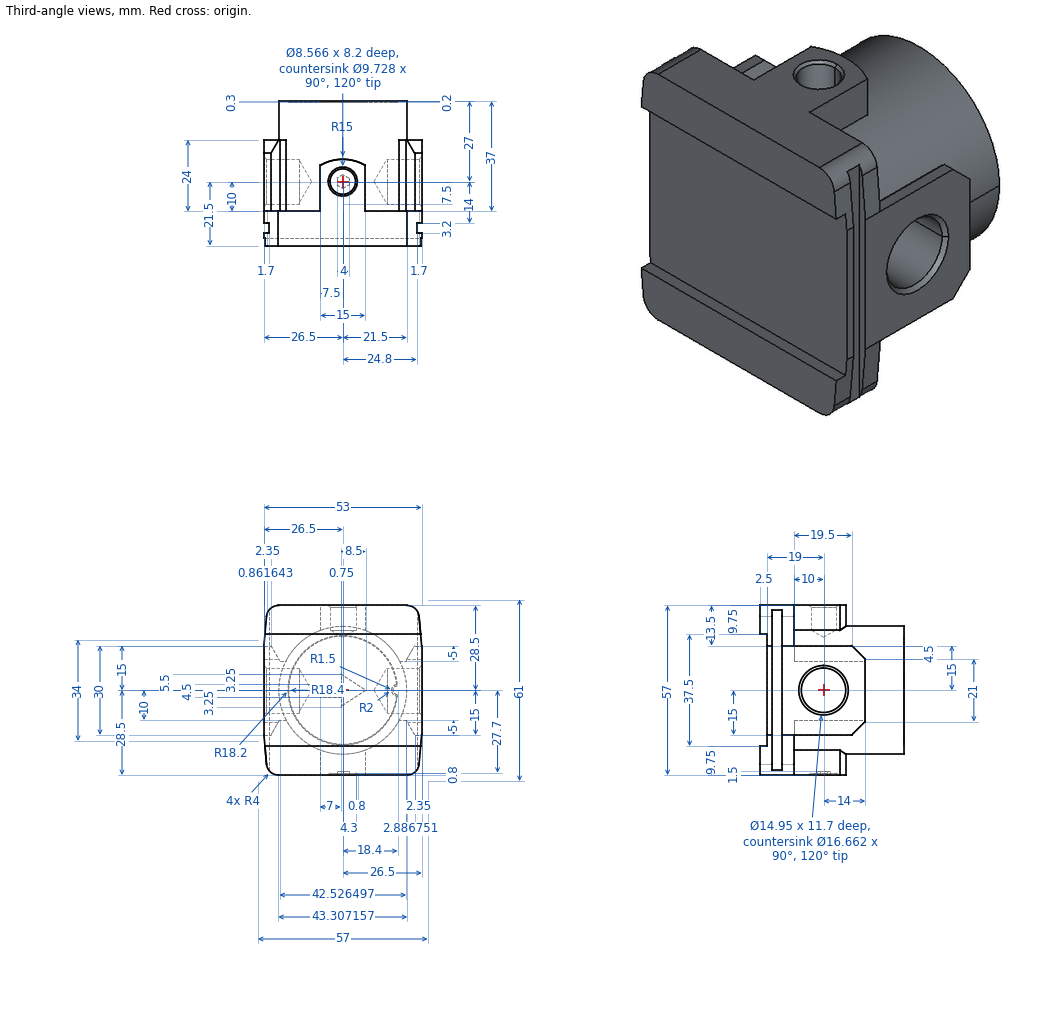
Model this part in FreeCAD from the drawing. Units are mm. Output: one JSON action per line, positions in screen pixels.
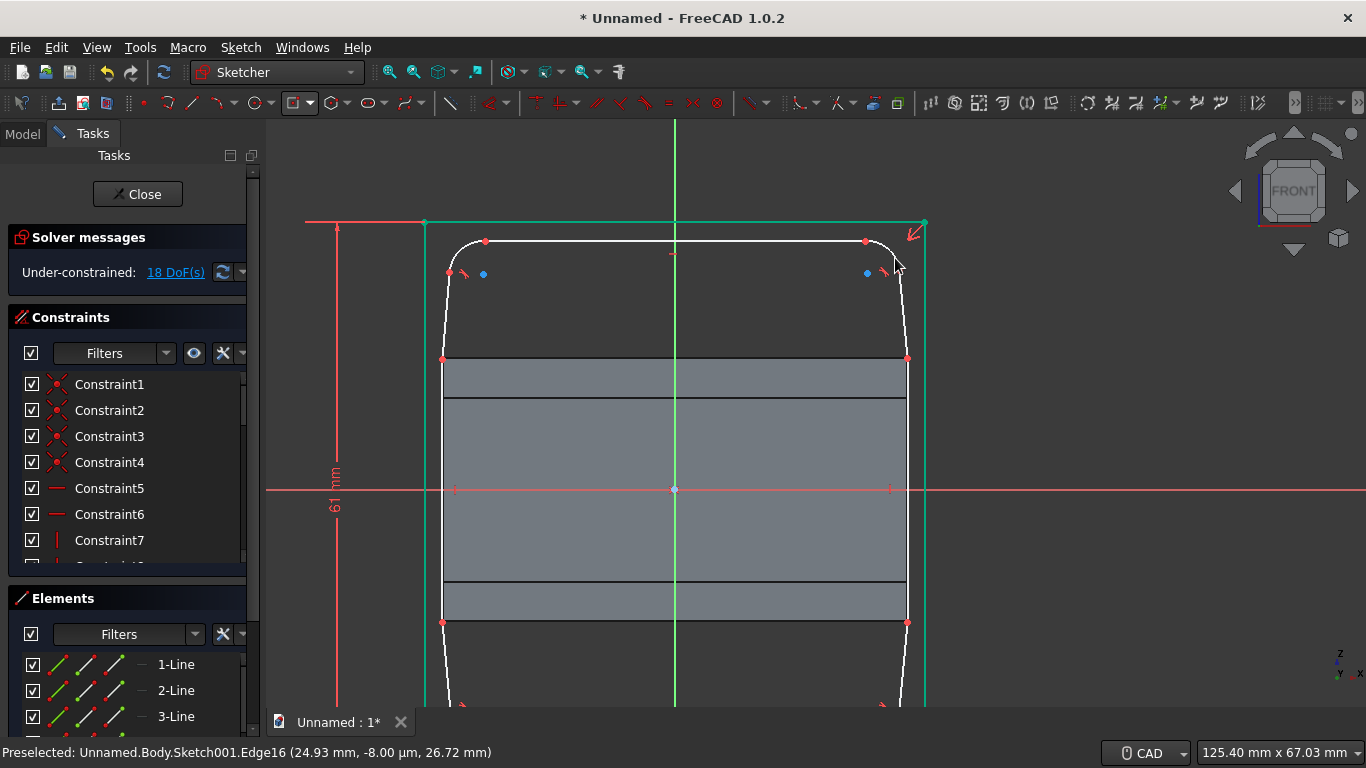
{"action": "left_click", "coordinate": [751, 241]}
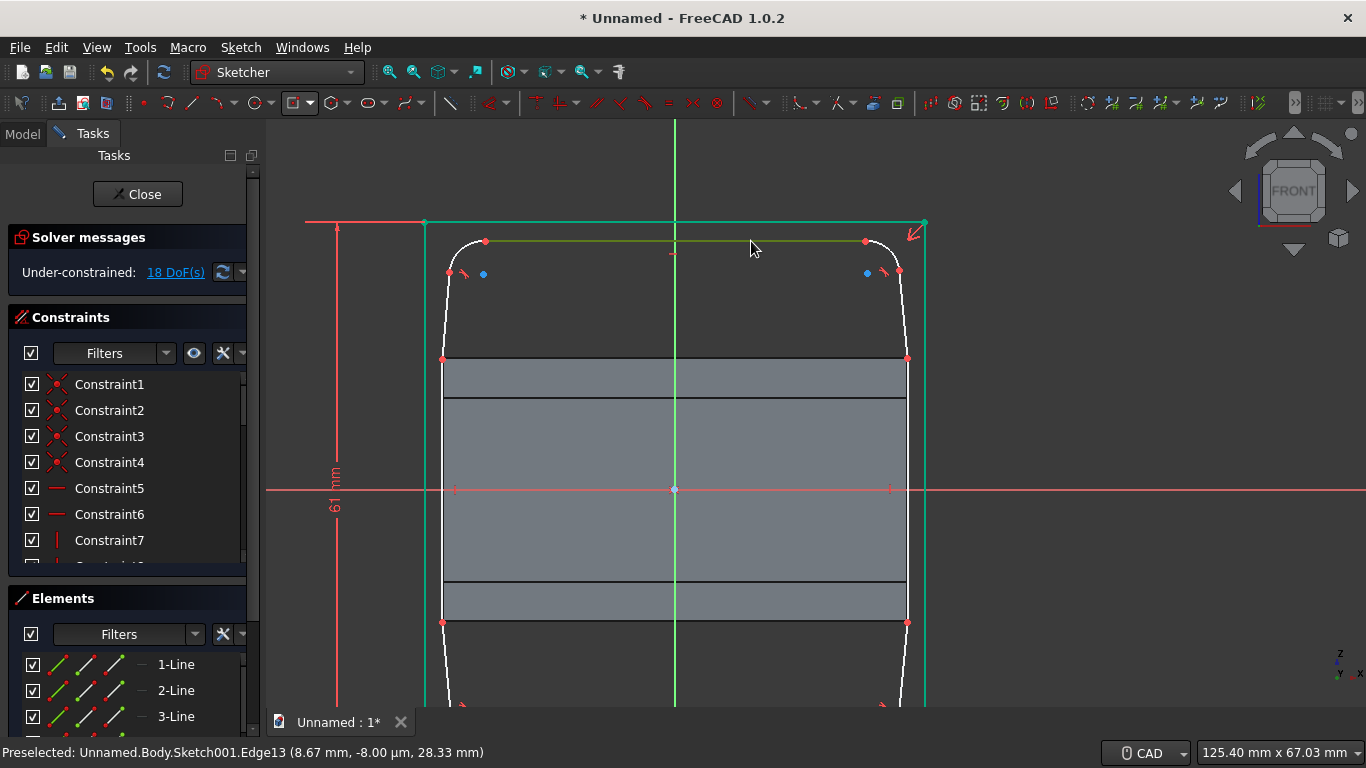
{"action": "left_click", "coordinate": [895, 256]}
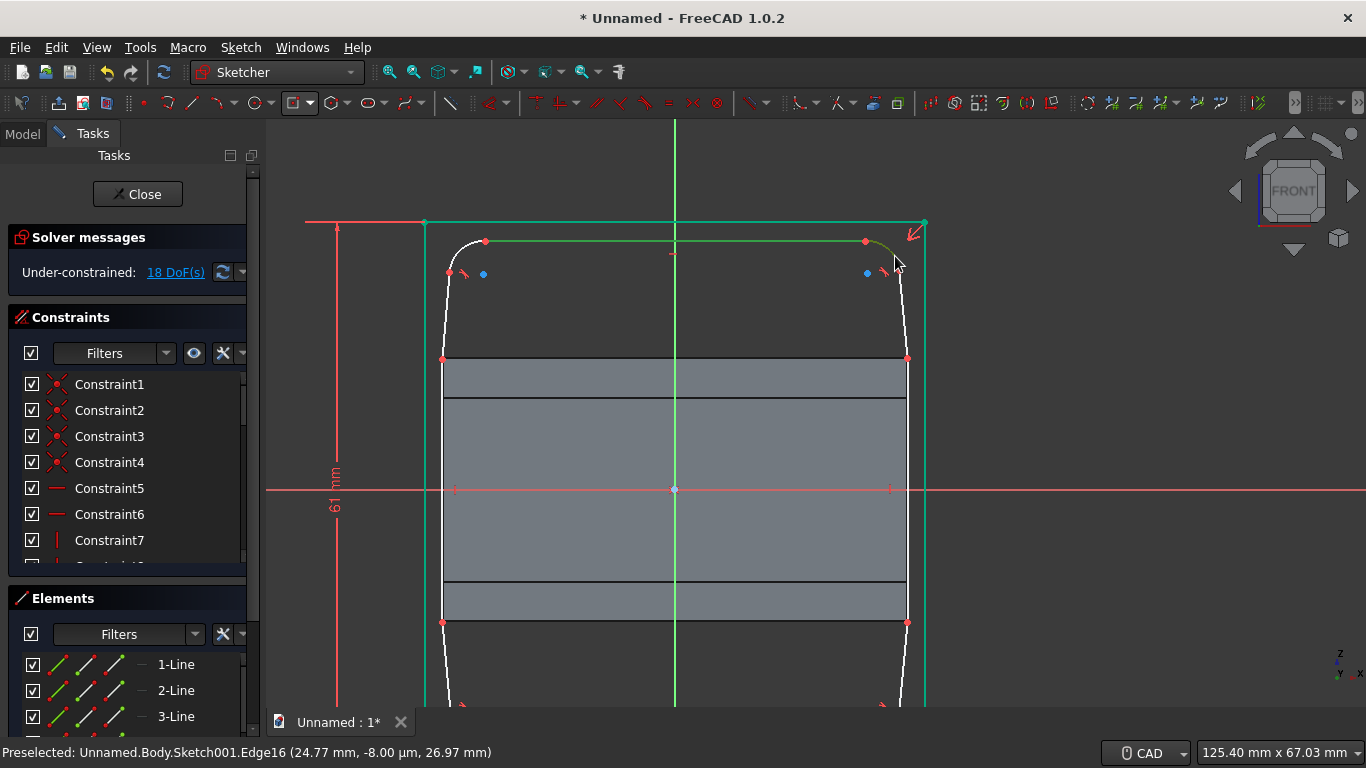
{"action": "left_click", "coordinate": [646, 104]}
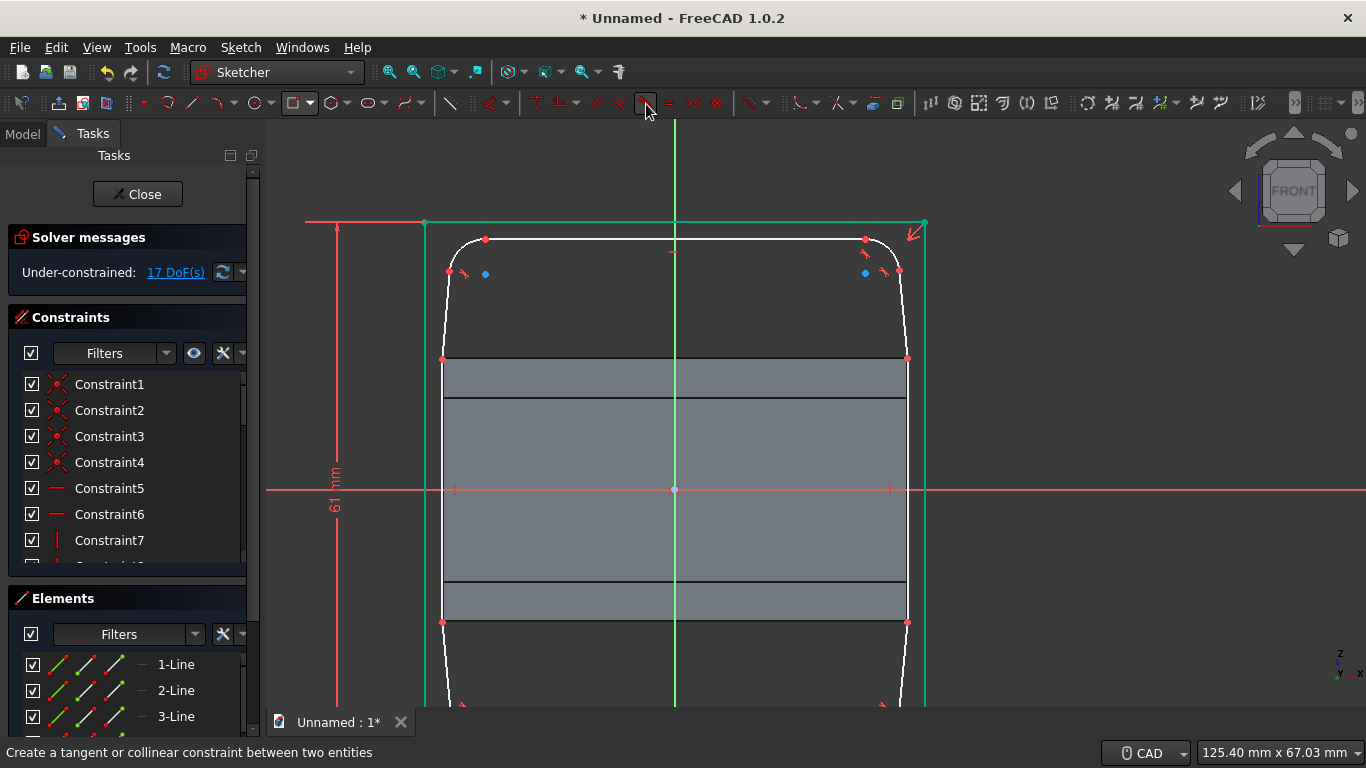
{"action": "left_click", "coordinate": [751, 239]}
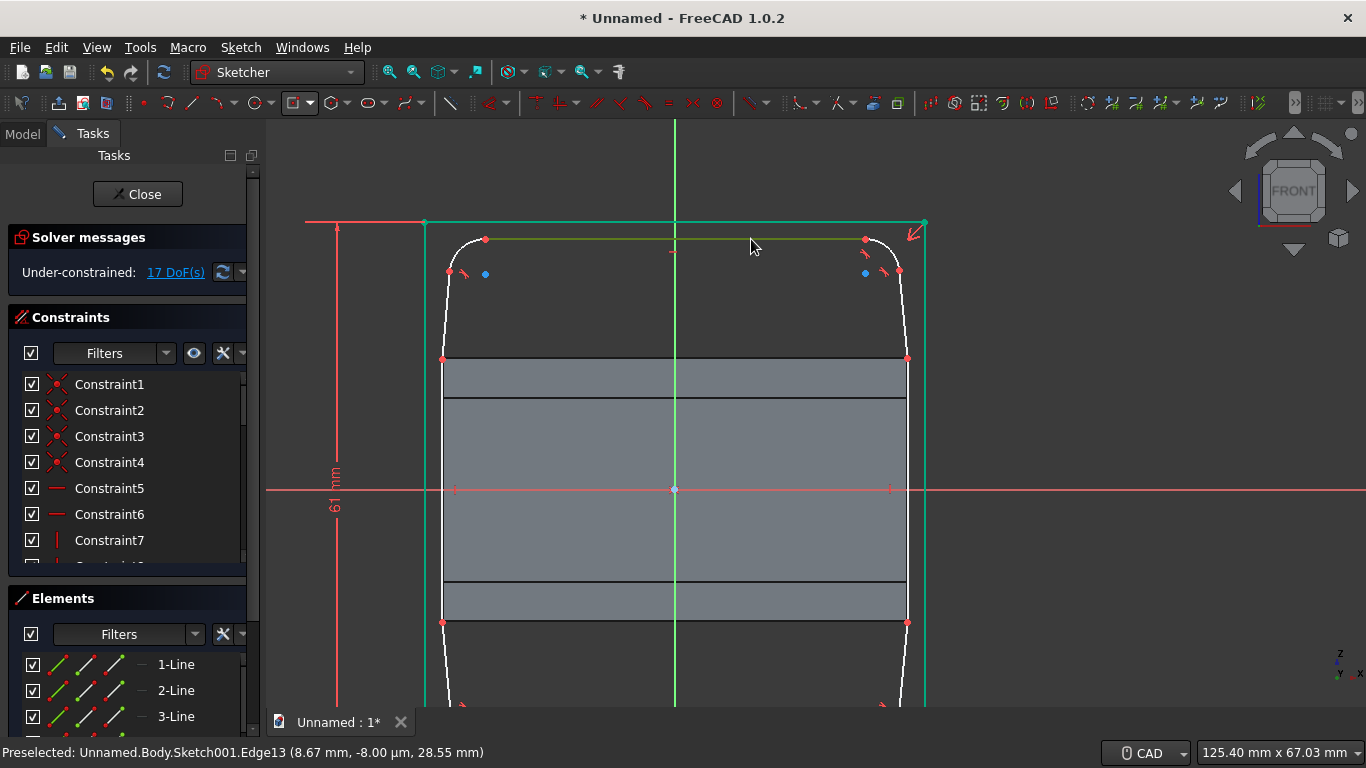
{"action": "left_click", "coordinate": [470, 243]}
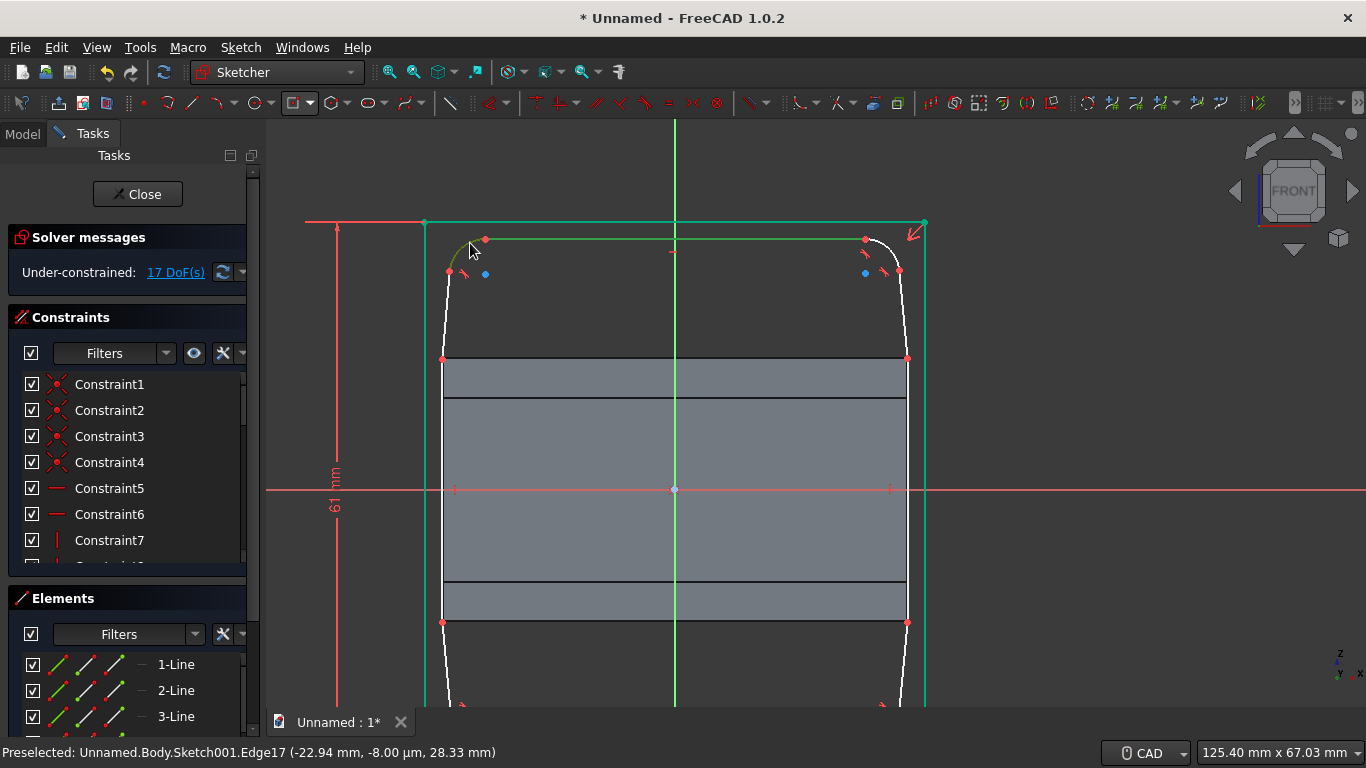
{"action": "key", "text": "t"}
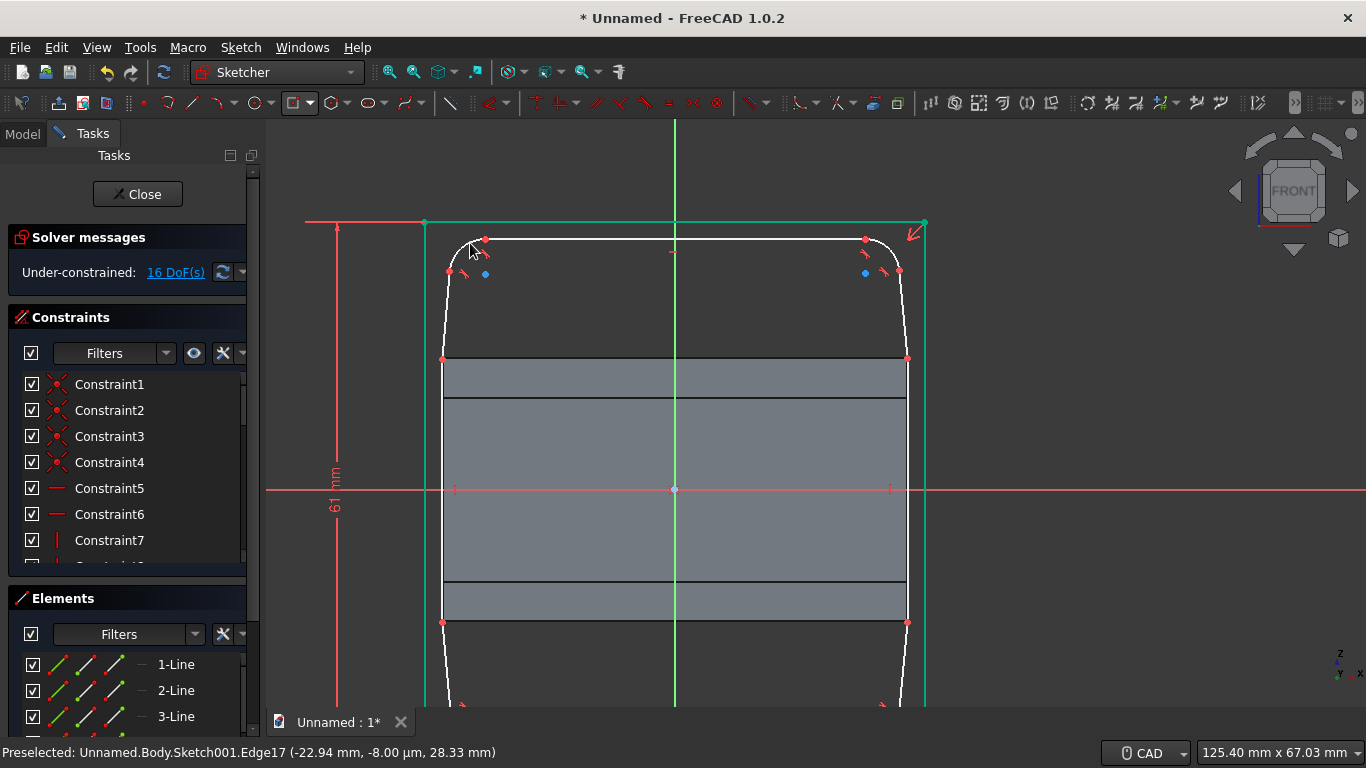
{"action": "scroll", "coordinate": [895, 257], "scroll_direction": "down", "scroll_amount": 2}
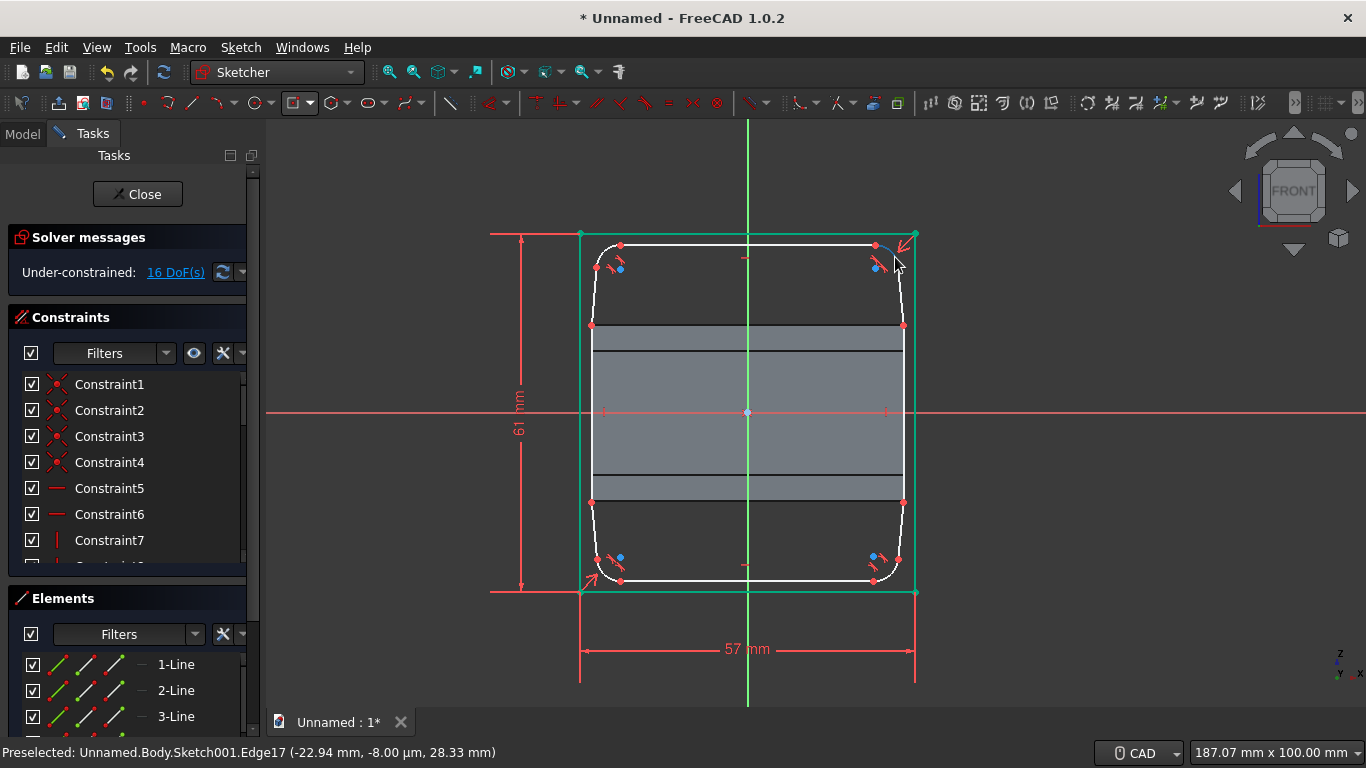
{"action": "scroll", "coordinate": [600, 570], "scroll_direction": "up", "scroll_amount": 2}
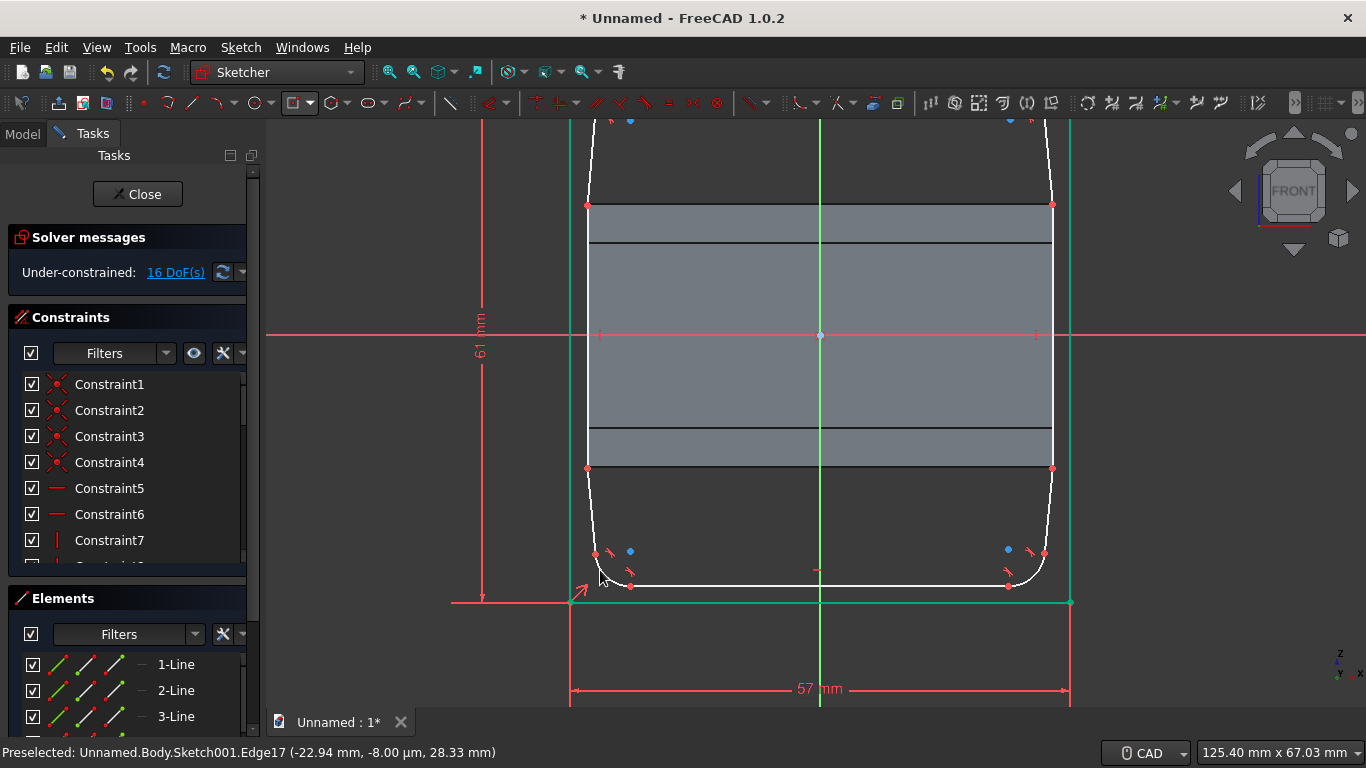
{"action": "left_click", "coordinate": [600, 569]}